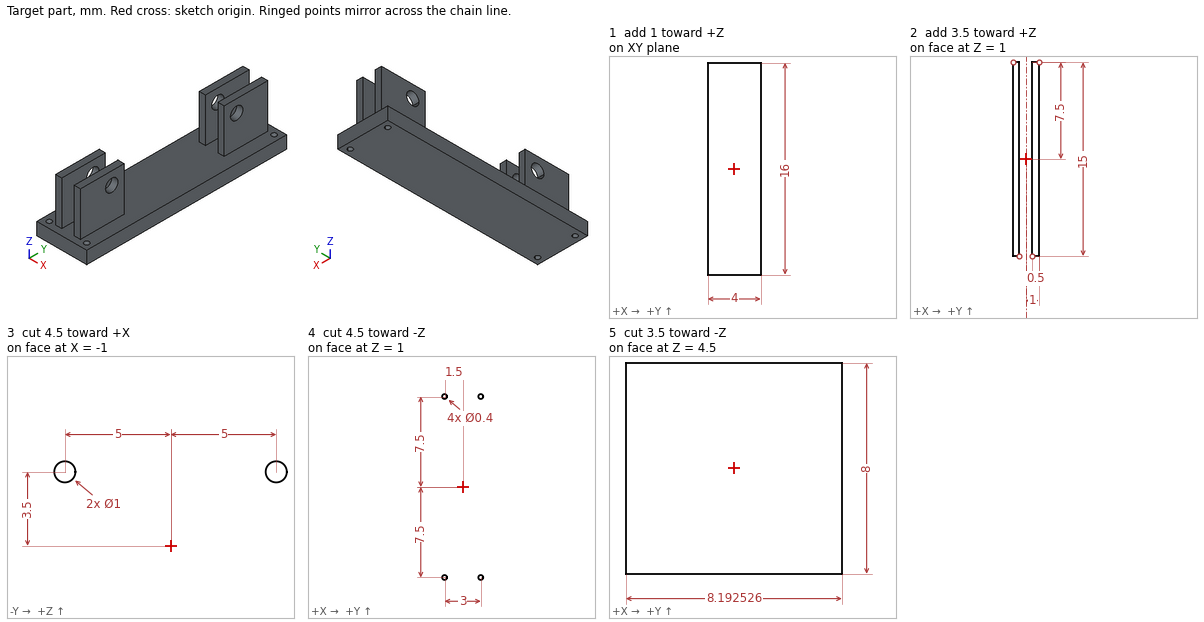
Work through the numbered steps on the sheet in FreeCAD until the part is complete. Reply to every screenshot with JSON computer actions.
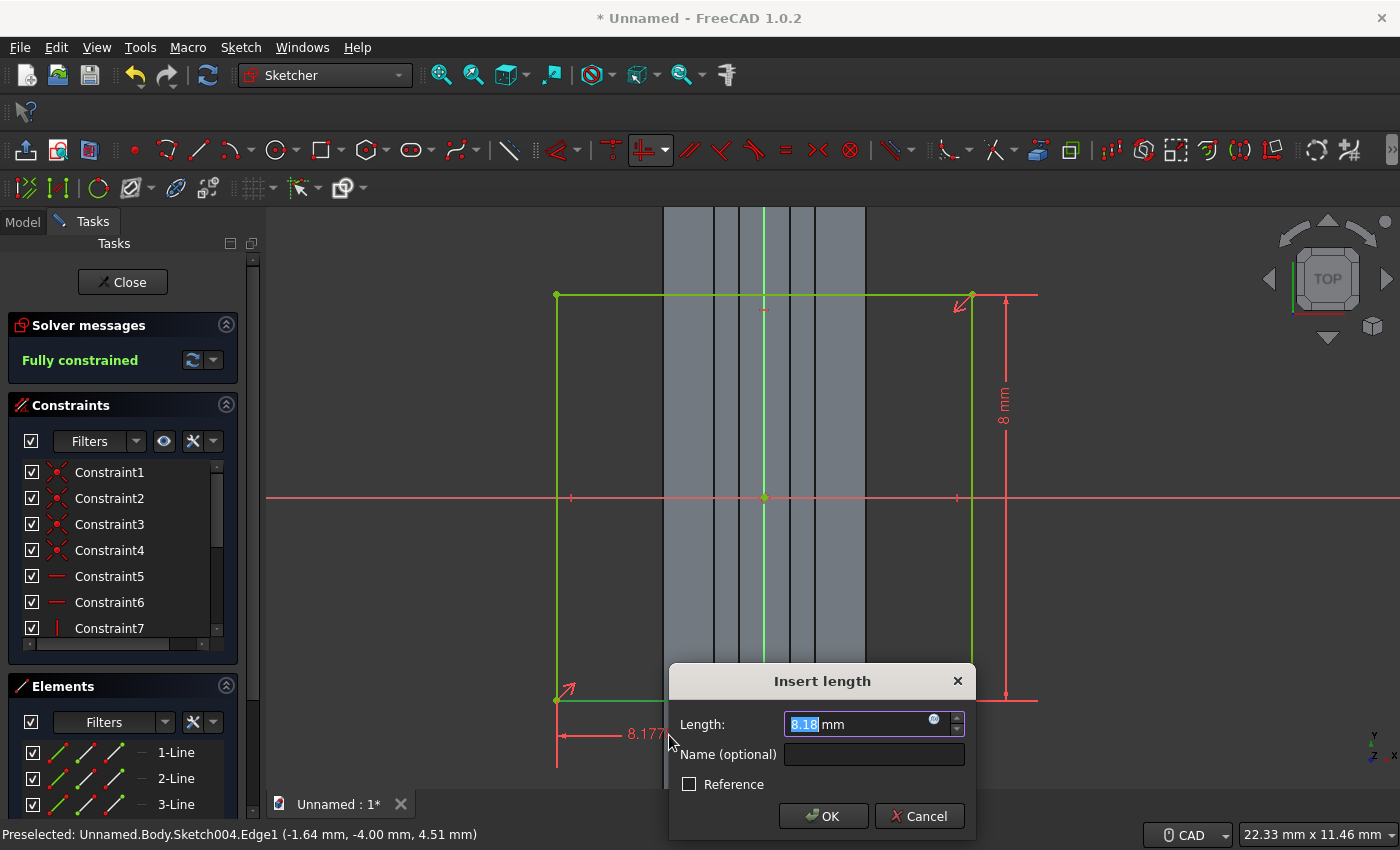
{"action": "type", "text": "8.192526"}
{"action": "key", "text": "Return"}
{"action": "key", "text": "Escape"}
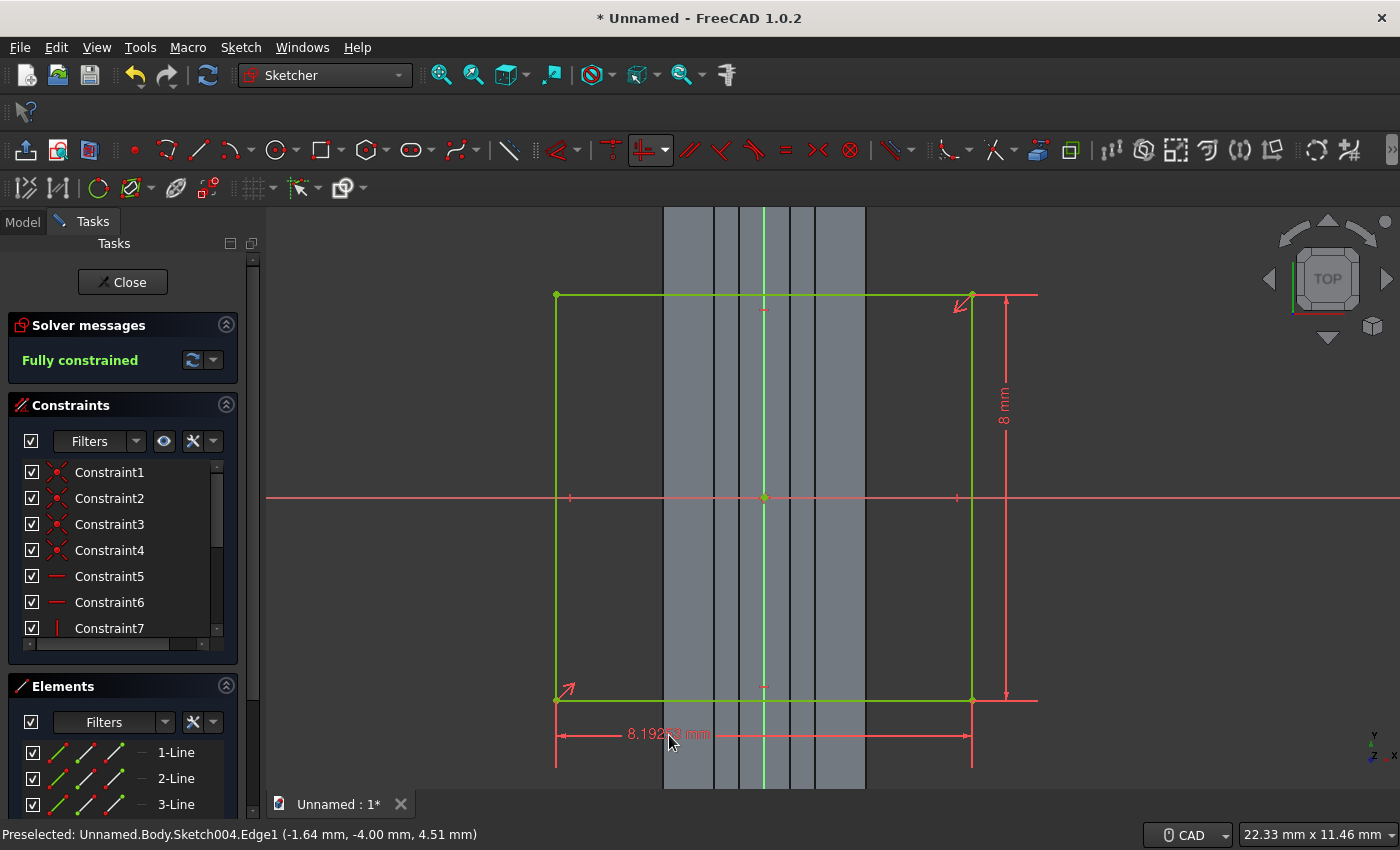
{"action": "left_click", "coordinate": [123, 282]}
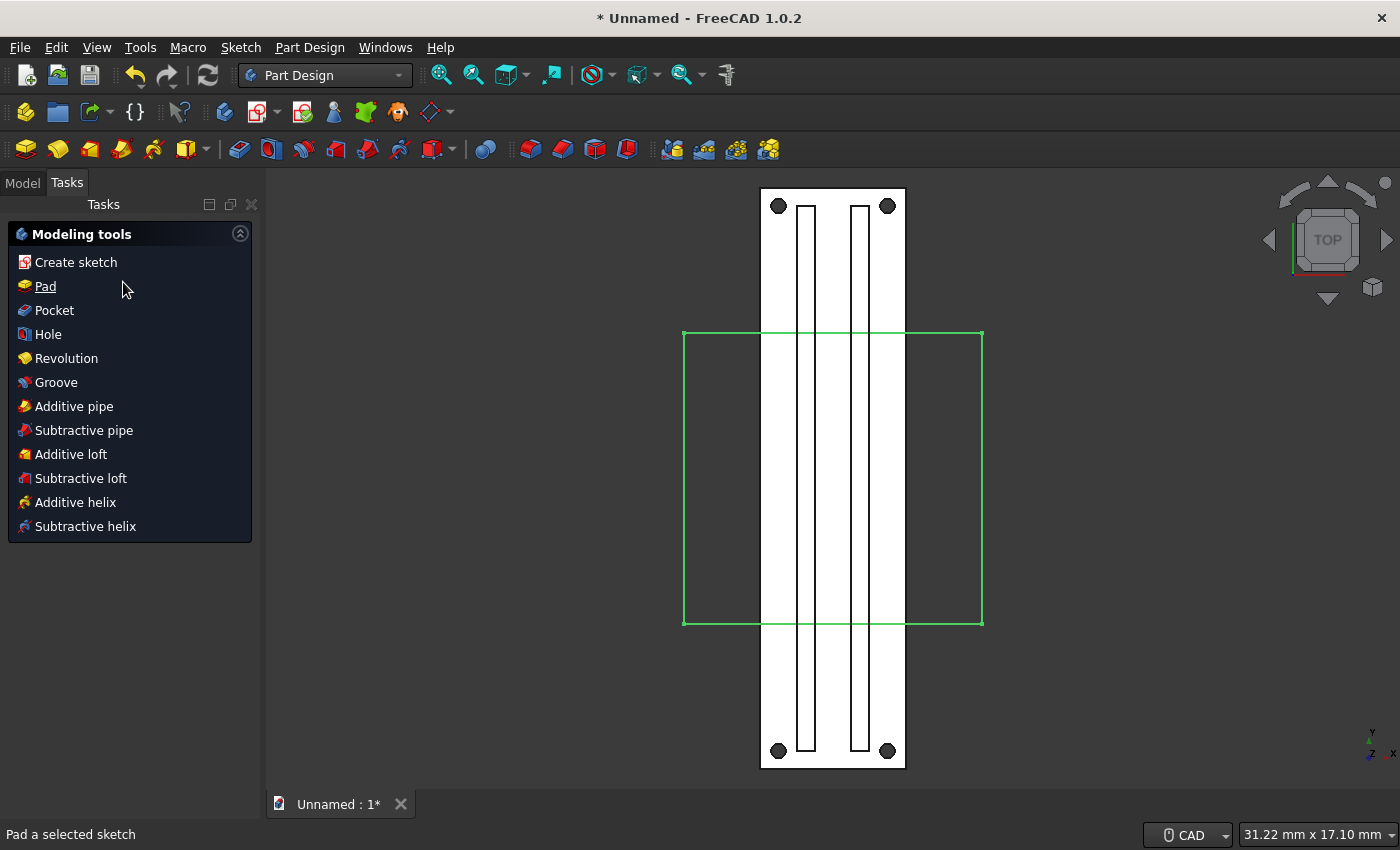
{"action": "left_click", "coordinate": [240, 150]}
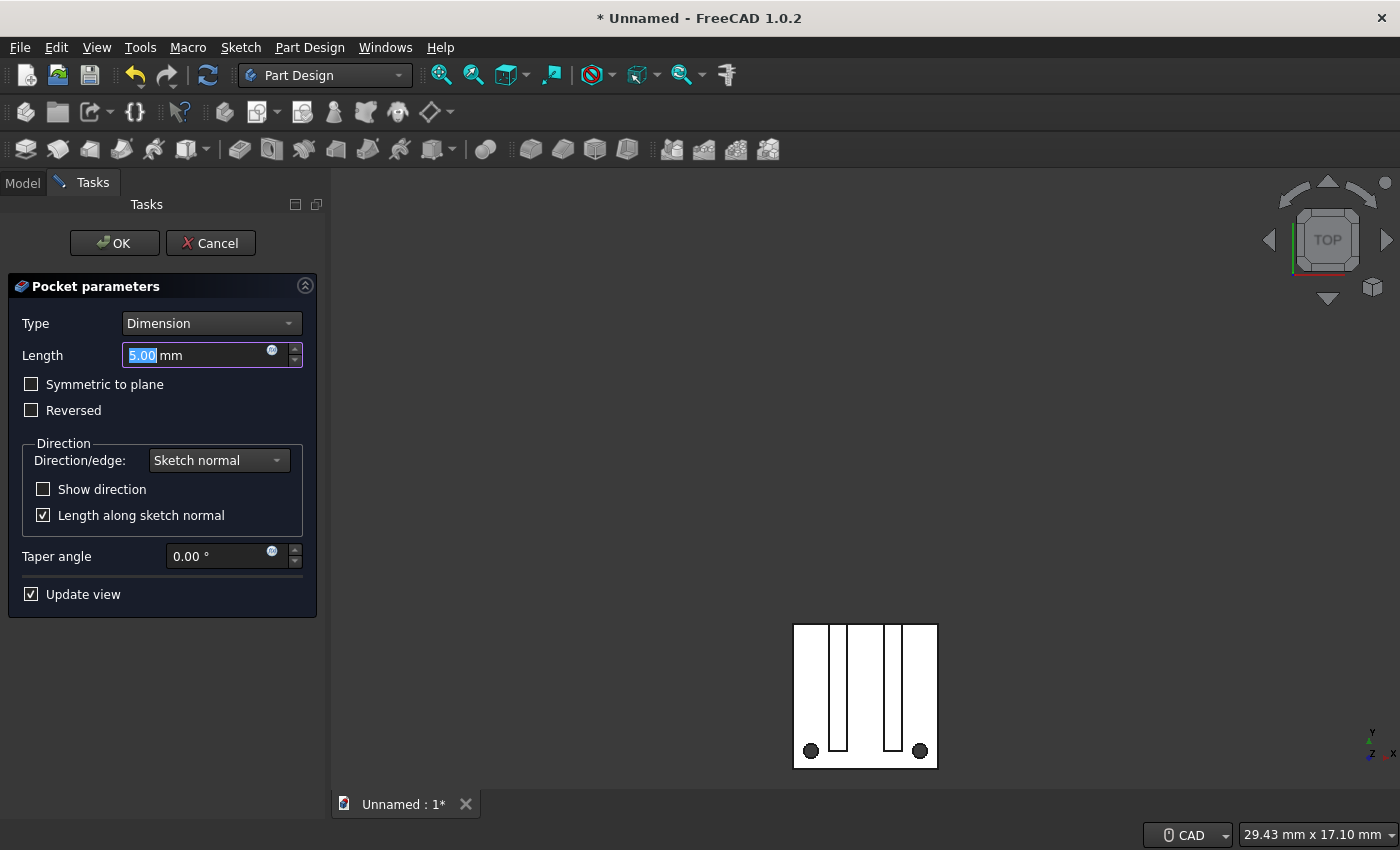
{"action": "type", "text": "3.5"}
{"action": "key", "text": "Tab"}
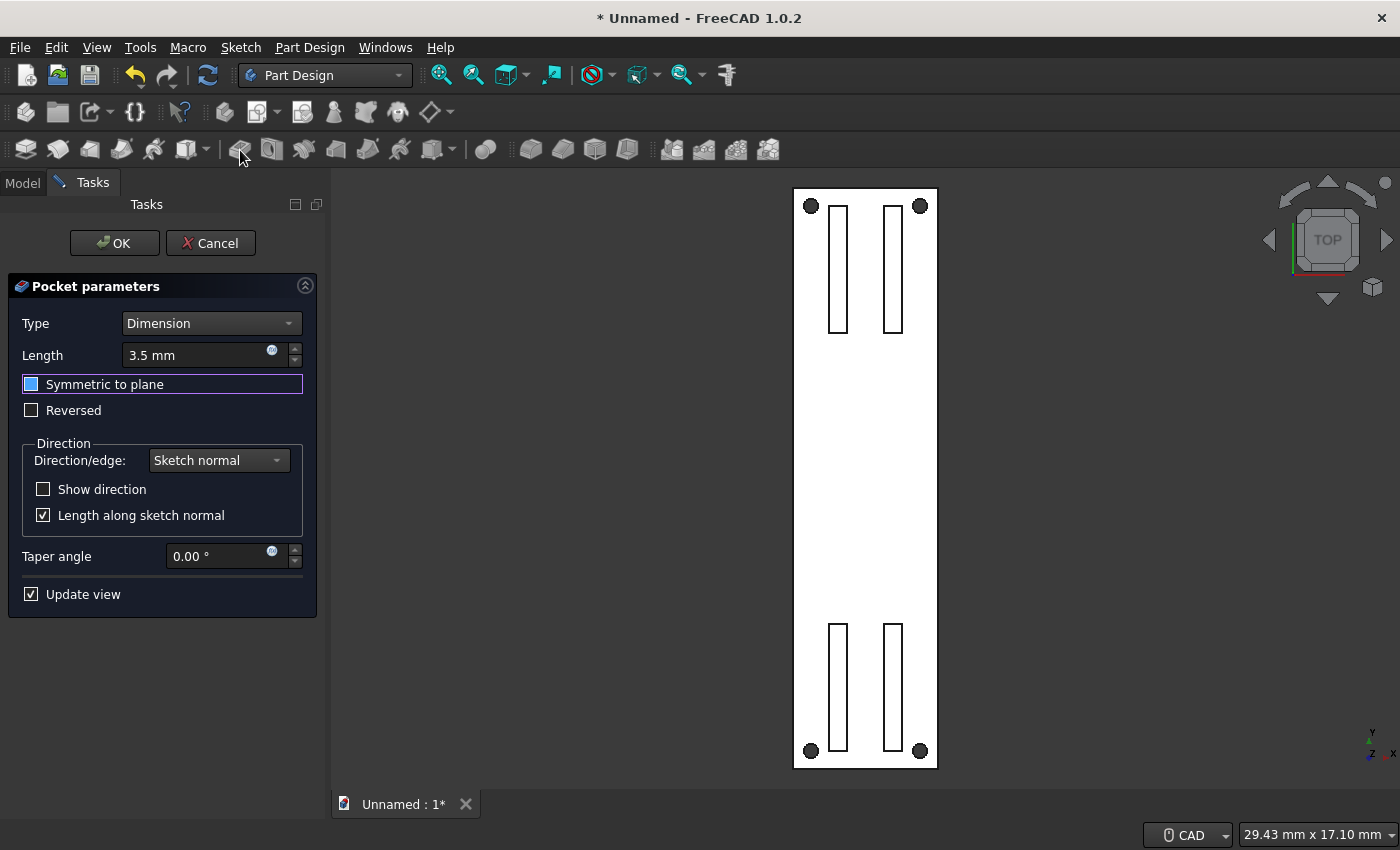
{"action": "left_click", "coordinate": [115, 243]}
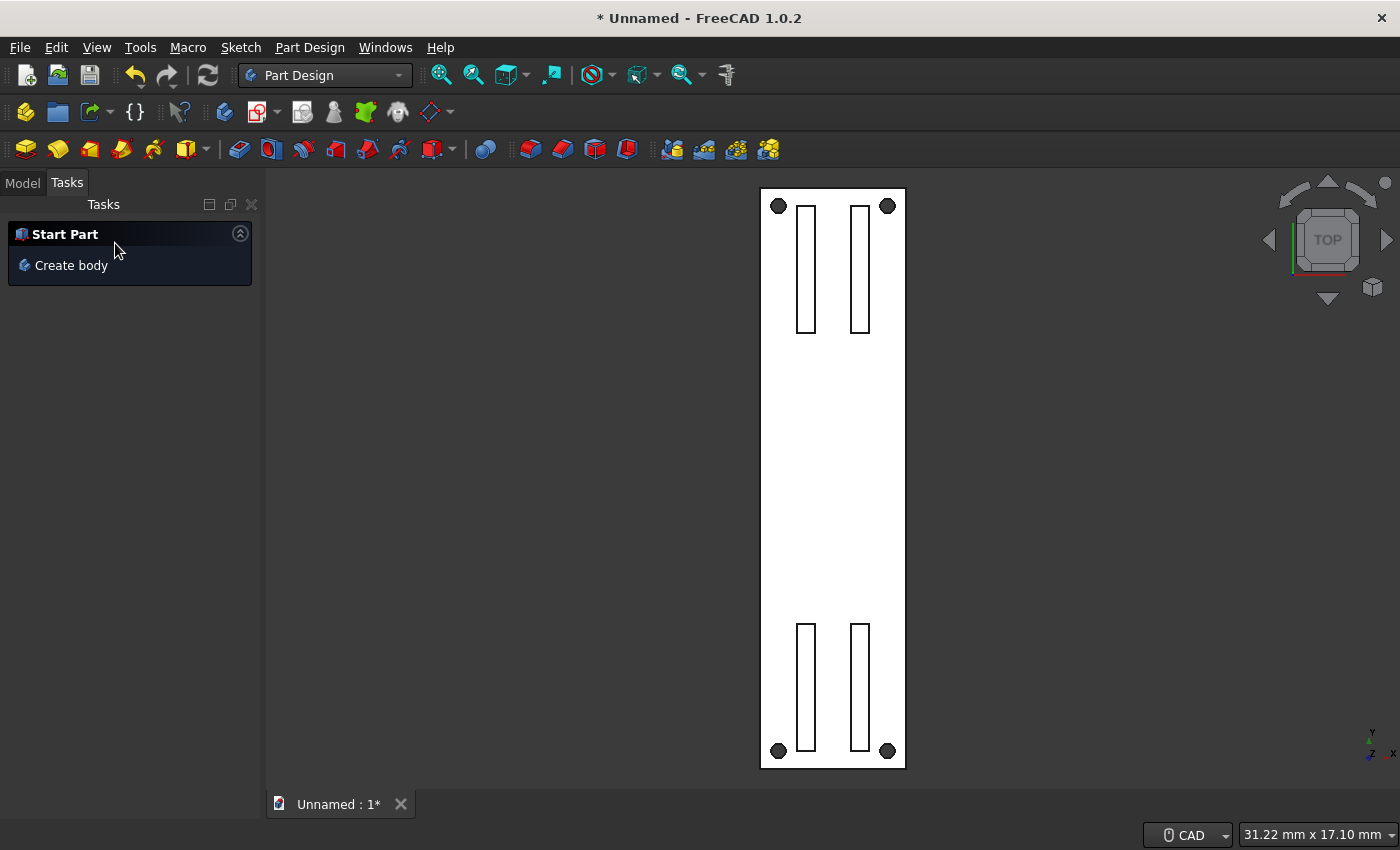
{"action": "key", "text": "0"}